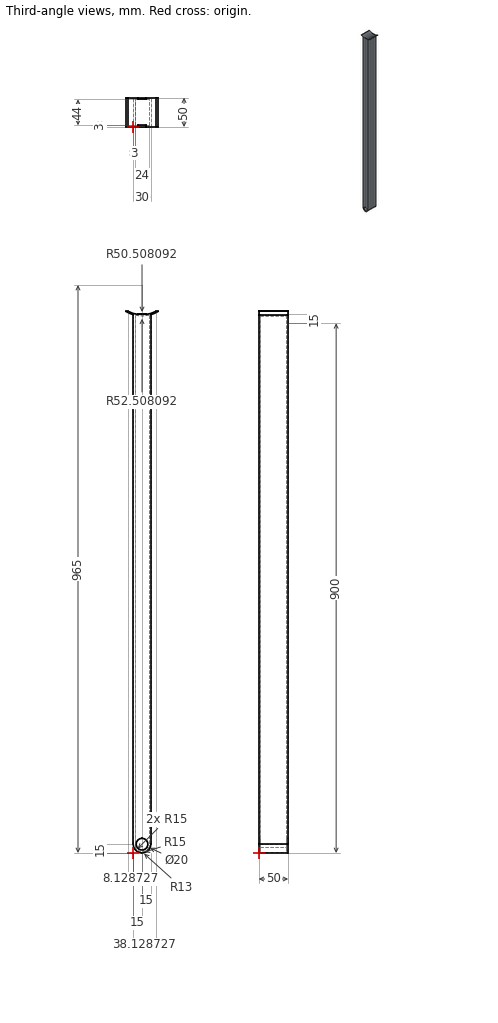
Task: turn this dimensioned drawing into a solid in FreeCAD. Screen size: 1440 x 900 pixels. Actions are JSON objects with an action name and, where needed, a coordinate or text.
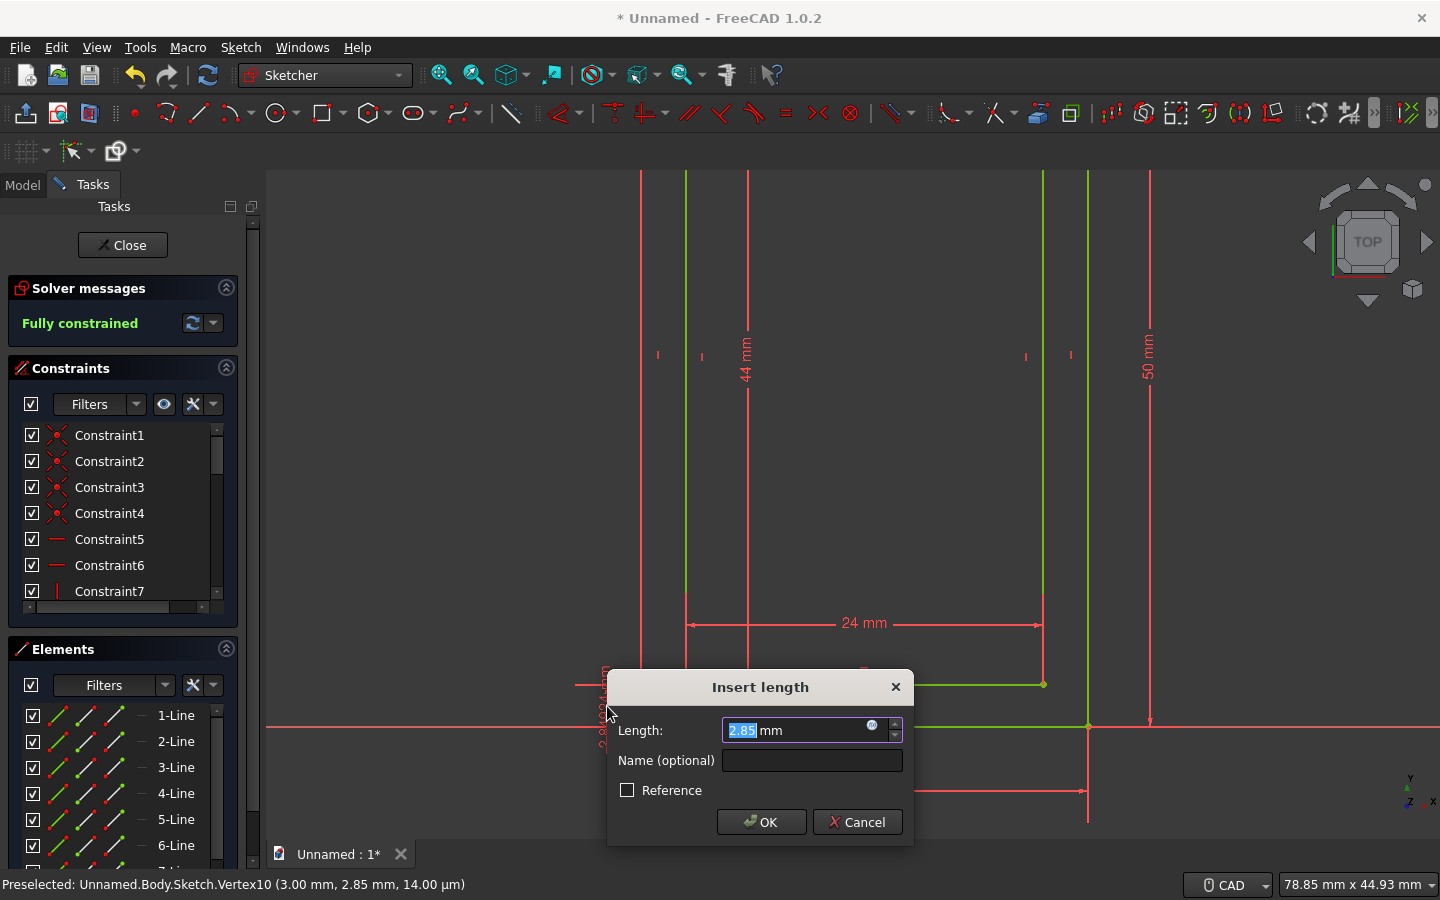
{"action": "type", "text": "3"}
{"action": "key", "text": "Return"}
{"action": "key", "text": "Escape"}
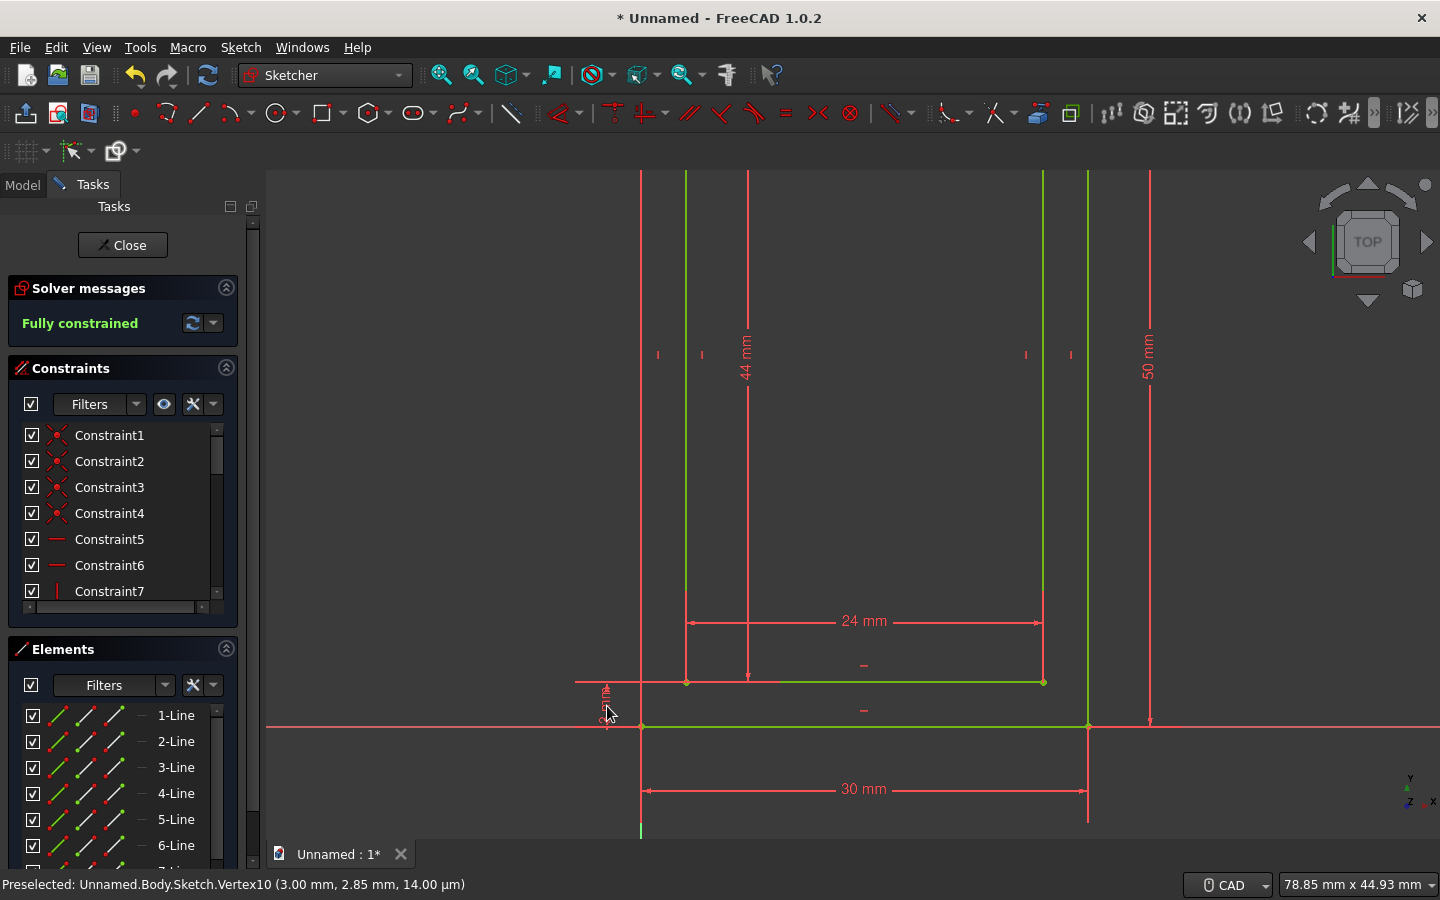
{"action": "left_click", "coordinate": [123, 245]}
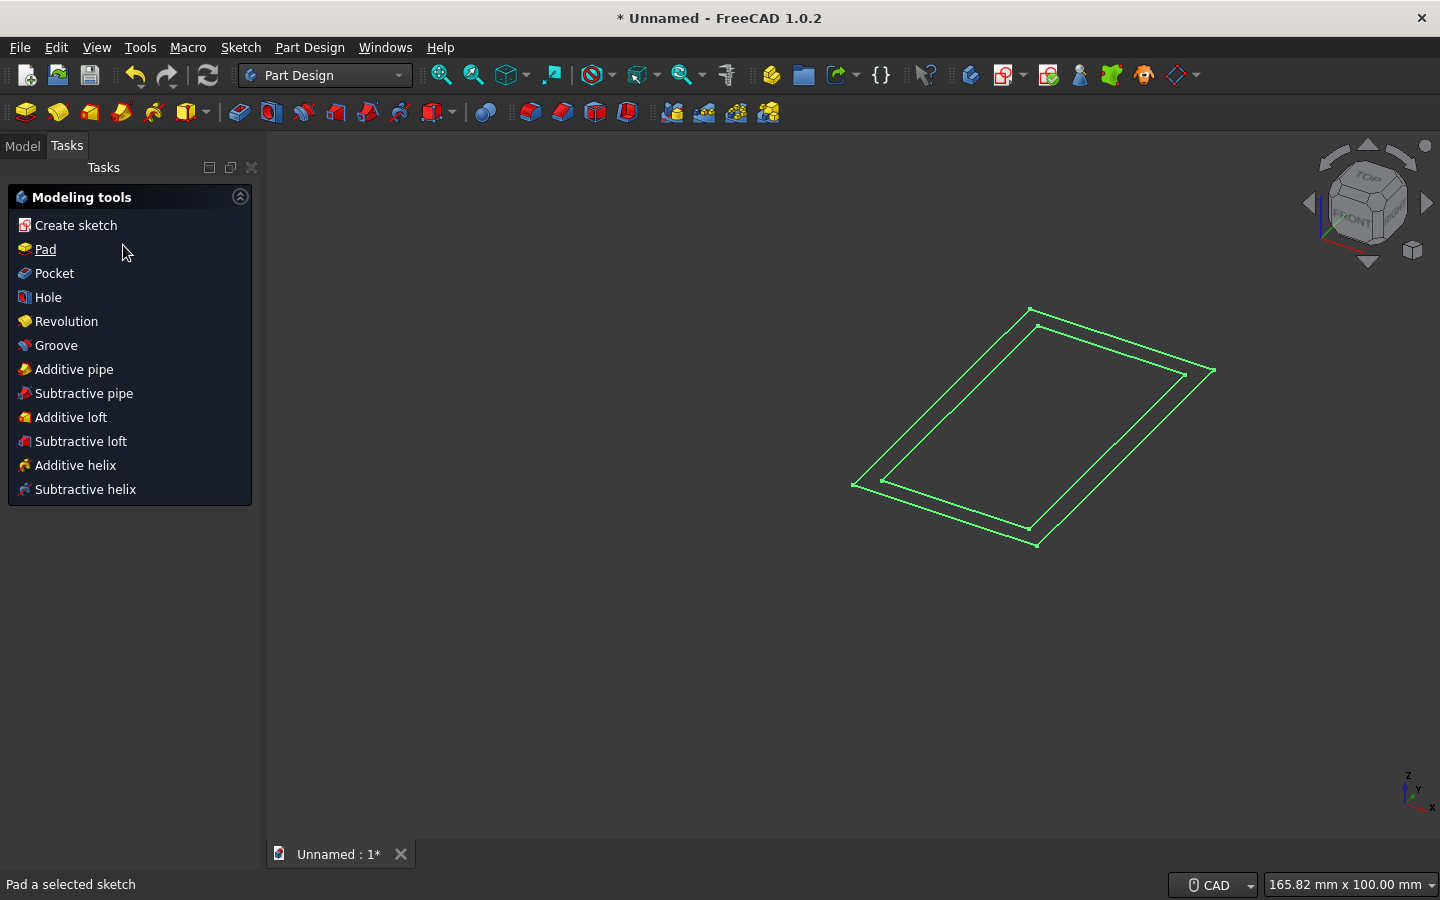
{"action": "left_click", "coordinate": [26, 112]}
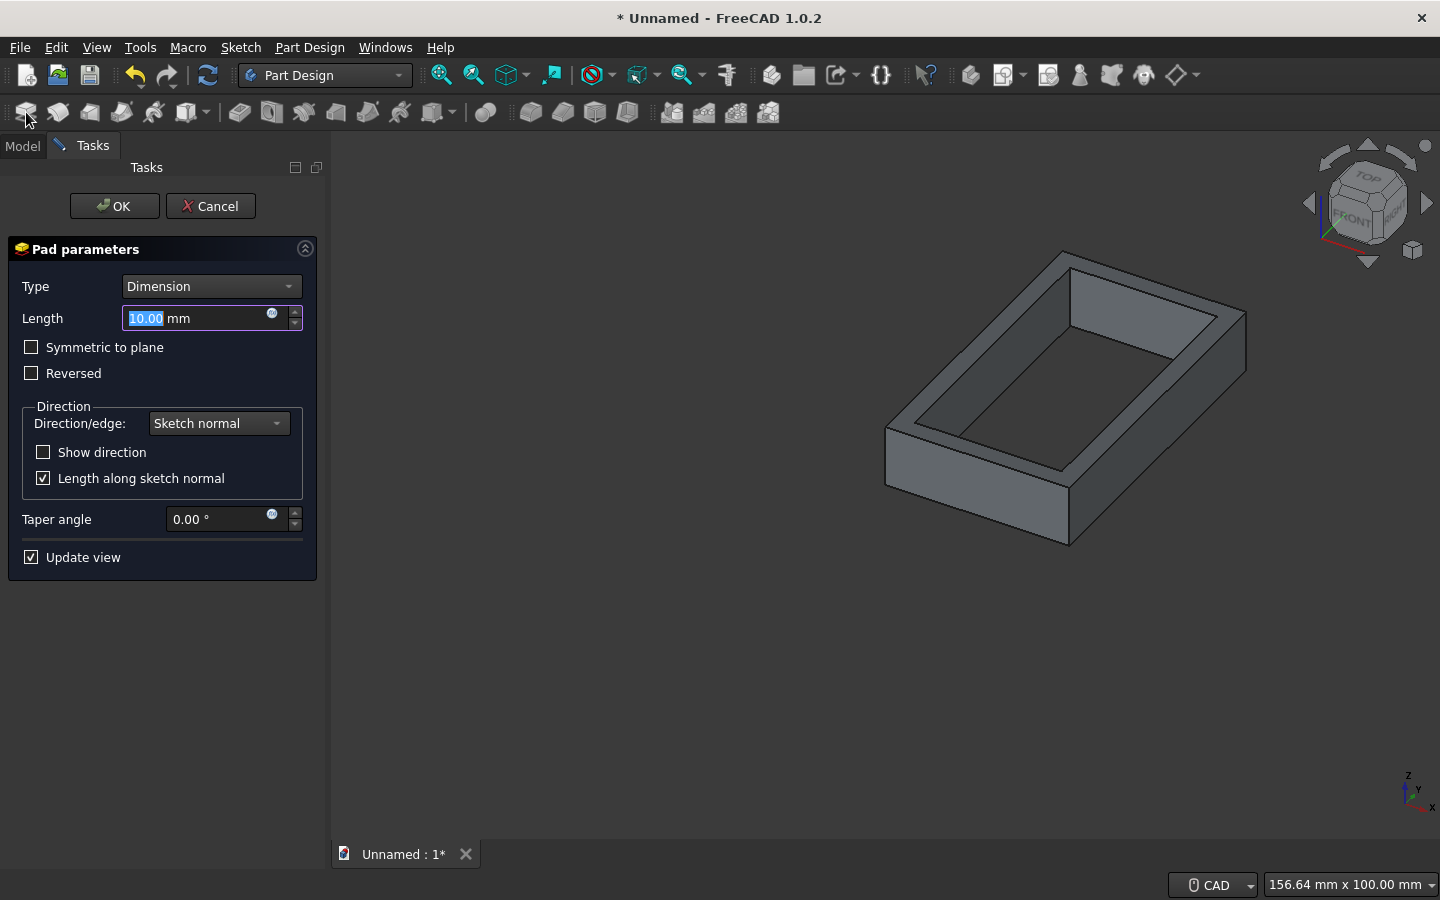
{"action": "type", "text": "900"}
{"action": "key", "text": "Tab"}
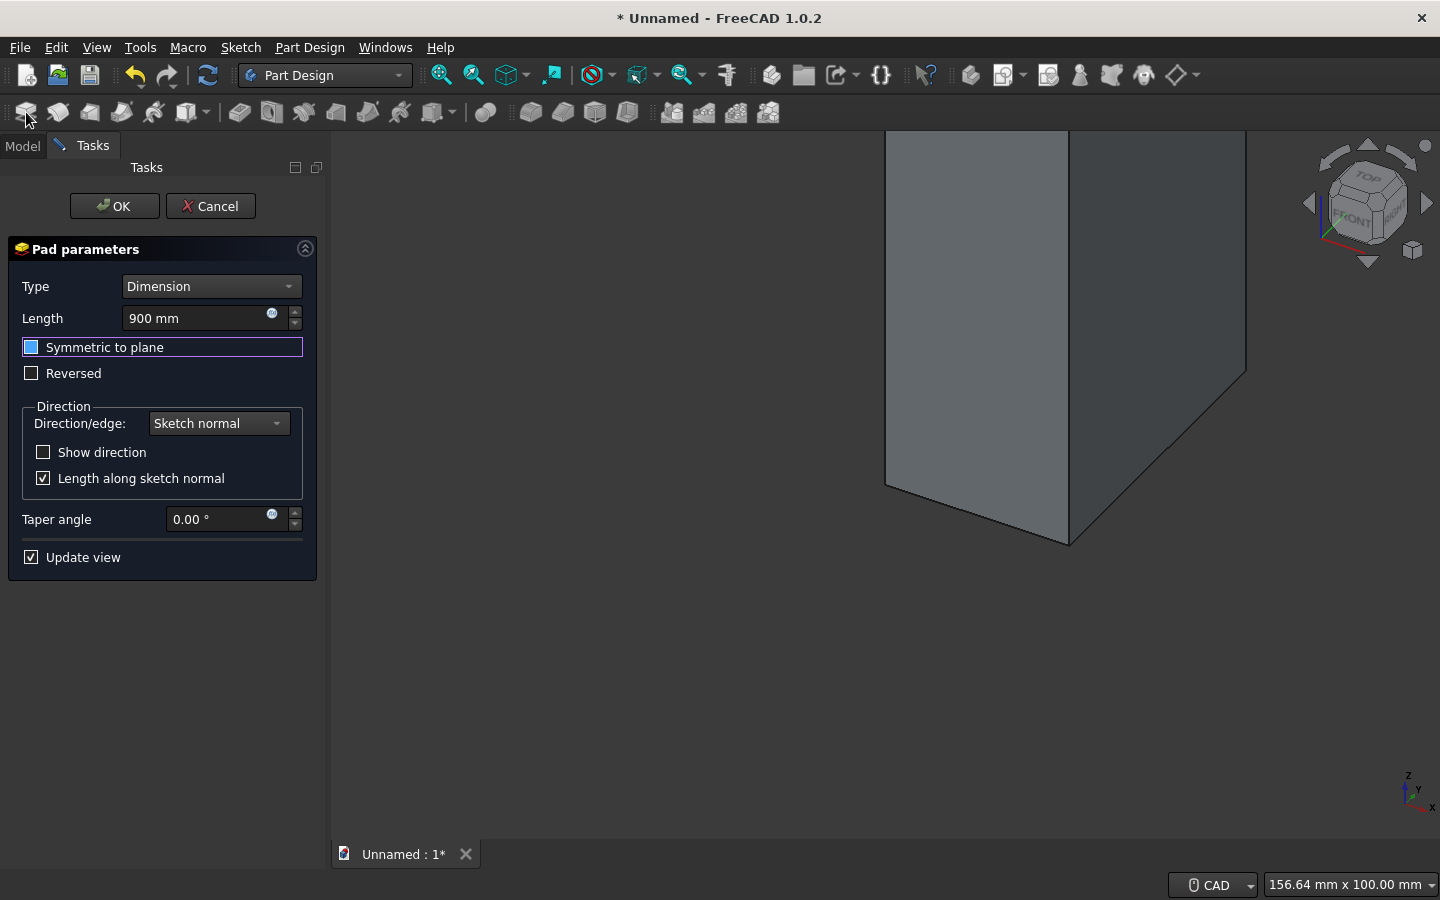
{"action": "left_click", "coordinate": [115, 206]}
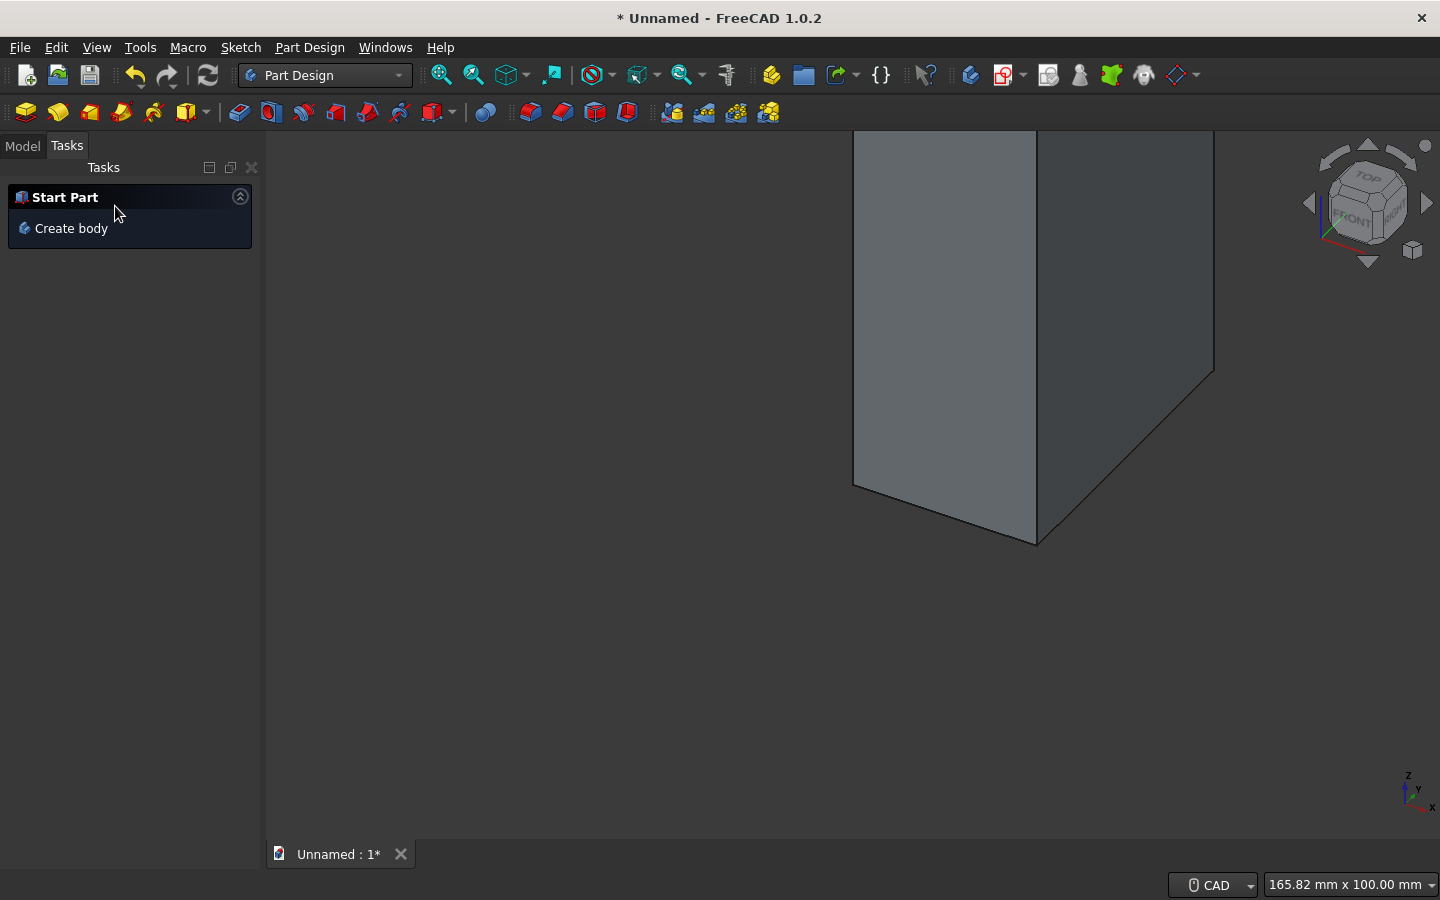
{"action": "left_click", "coordinate": [442, 76]}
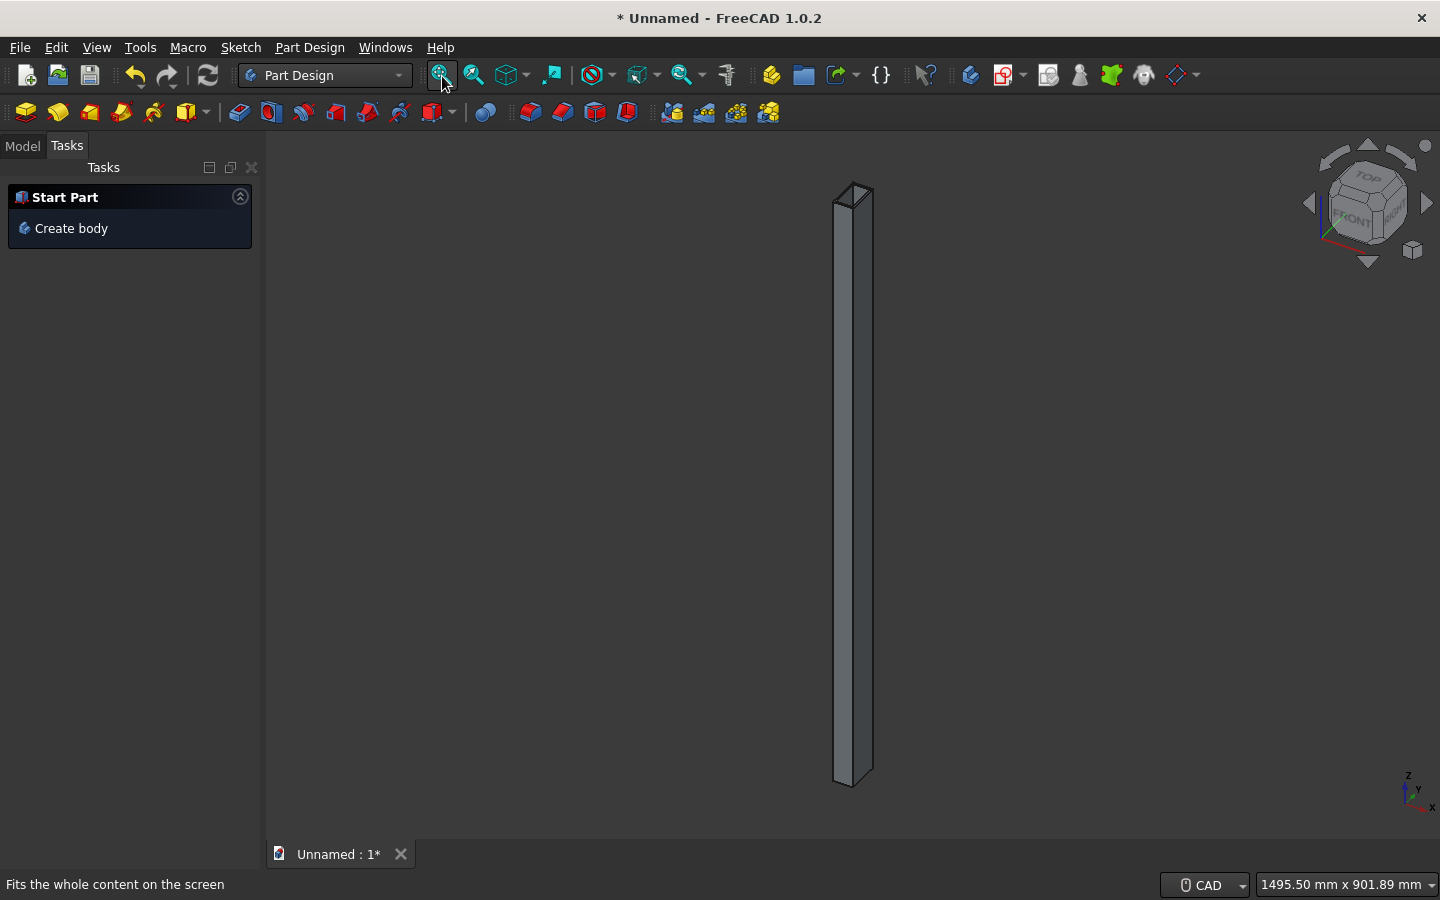
{"action": "key", "text": "4"}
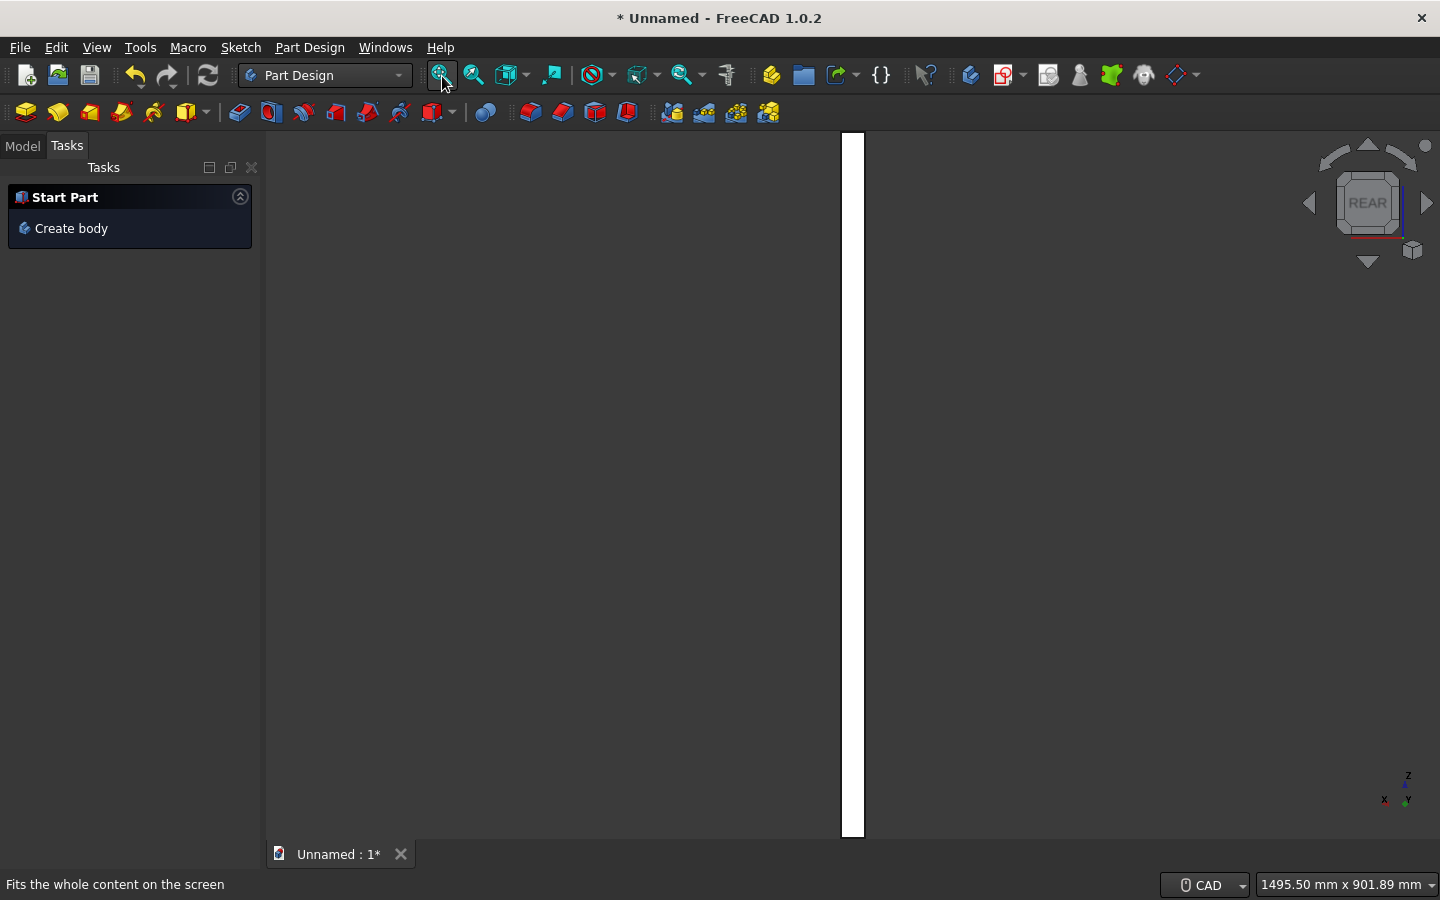
{"action": "left_click", "coordinate": [853, 181]}